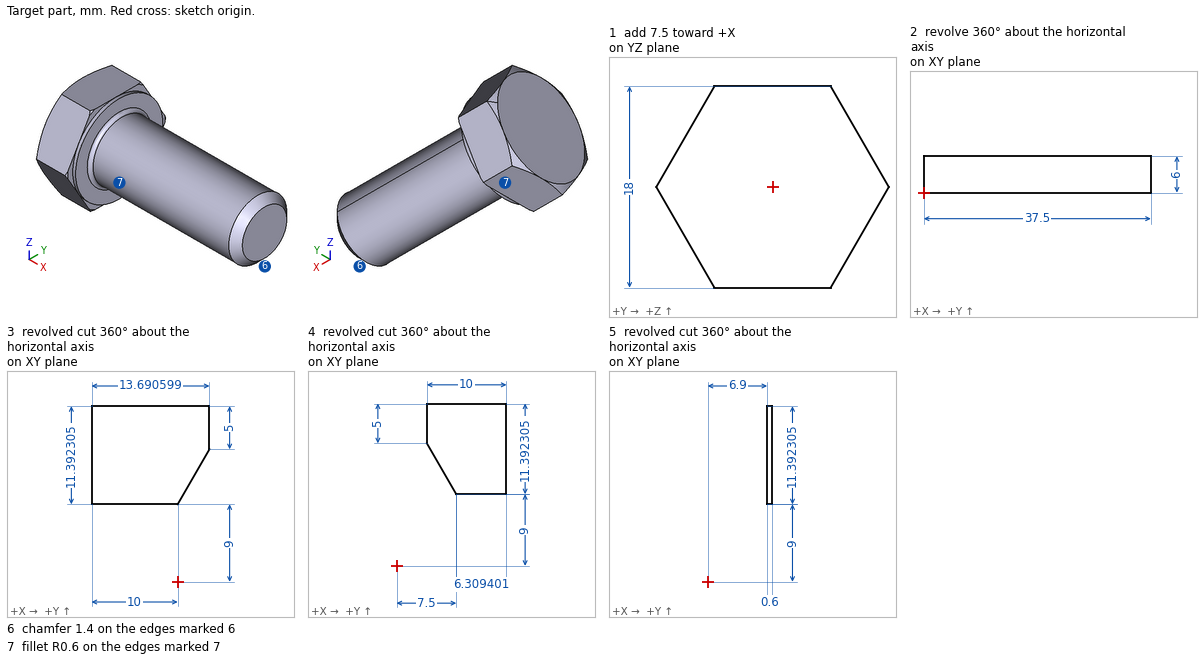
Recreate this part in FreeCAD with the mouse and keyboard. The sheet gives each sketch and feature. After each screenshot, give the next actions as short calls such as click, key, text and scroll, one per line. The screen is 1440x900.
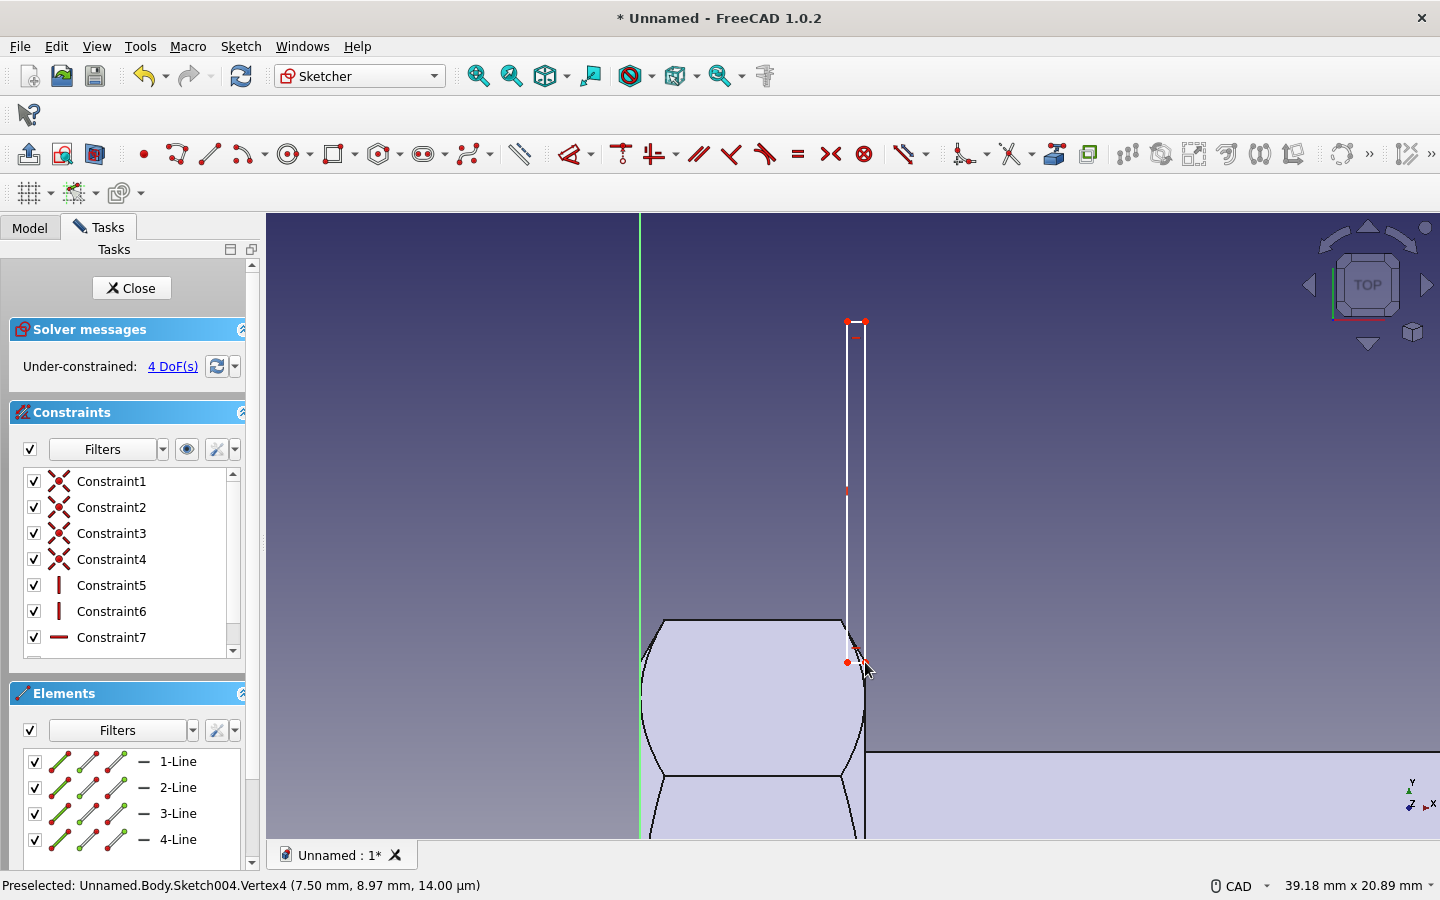
key(d)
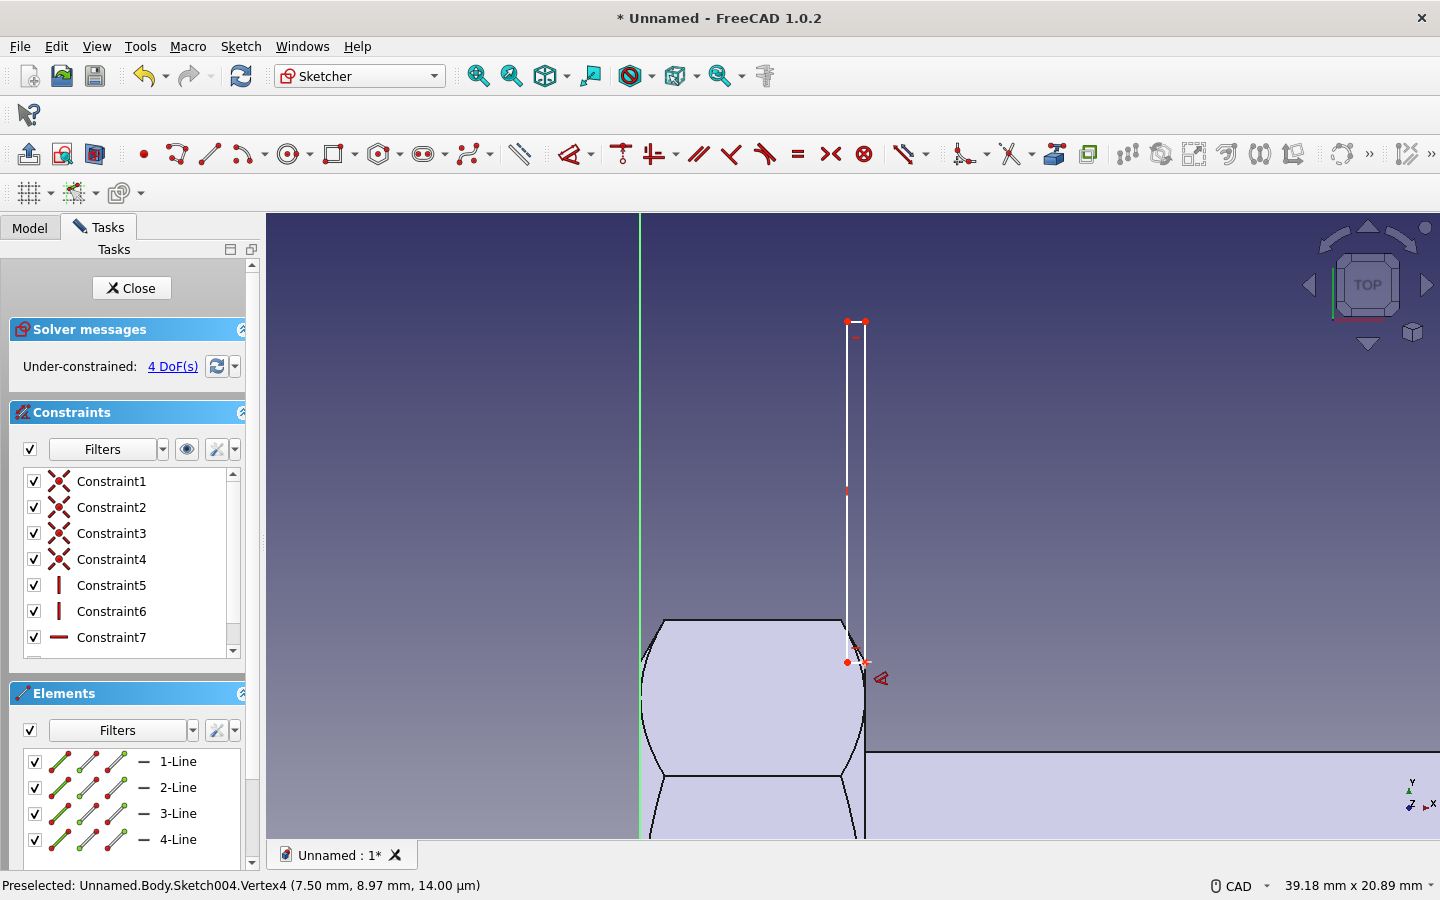
click(847, 663)
click(606, 737)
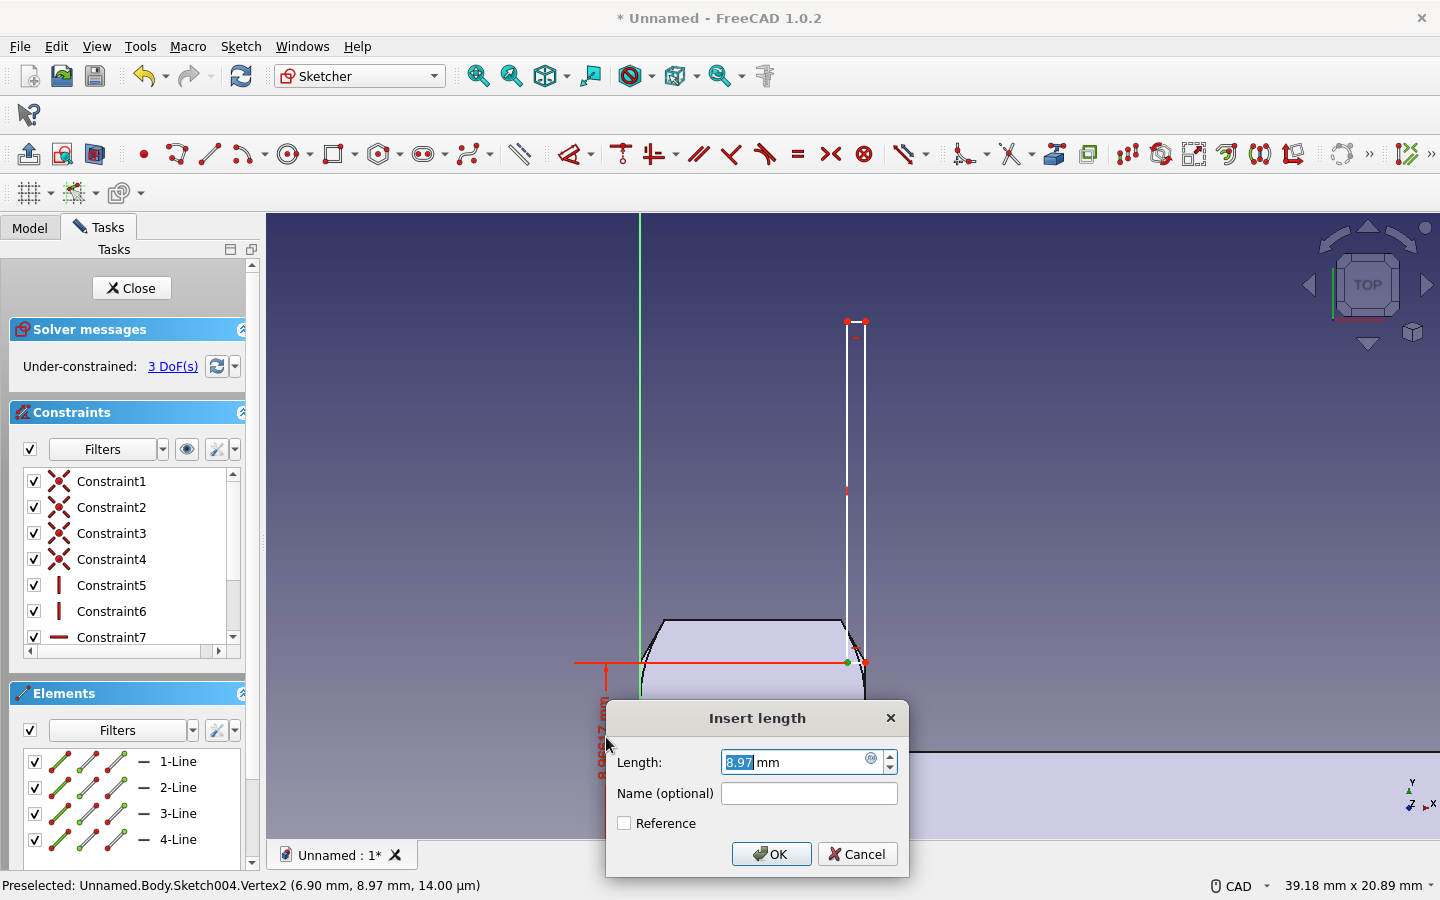
text(9)
key(Return)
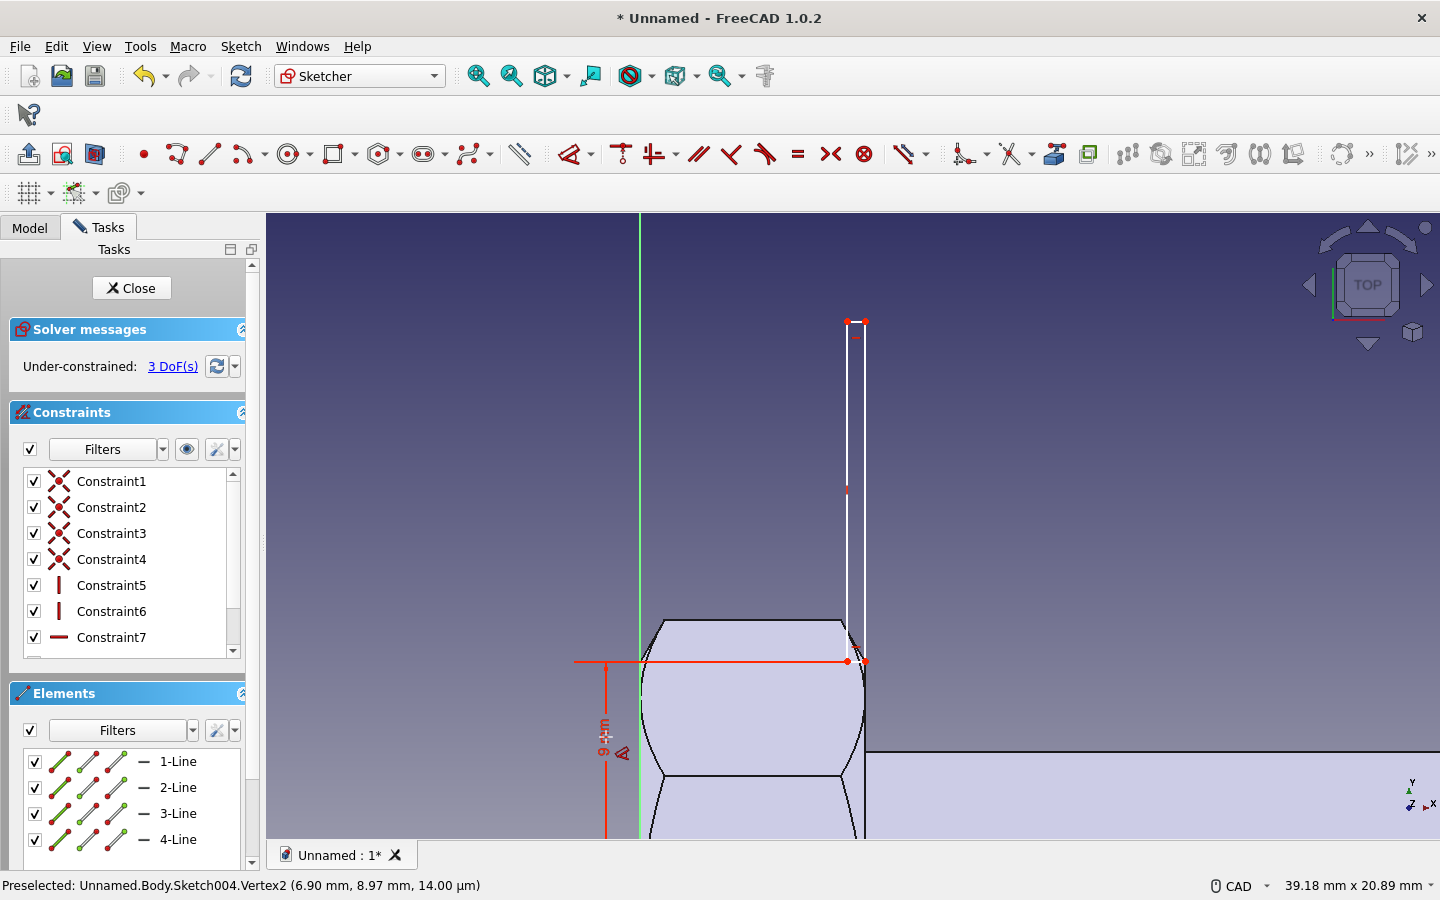
scroll(856, 662, up, 4)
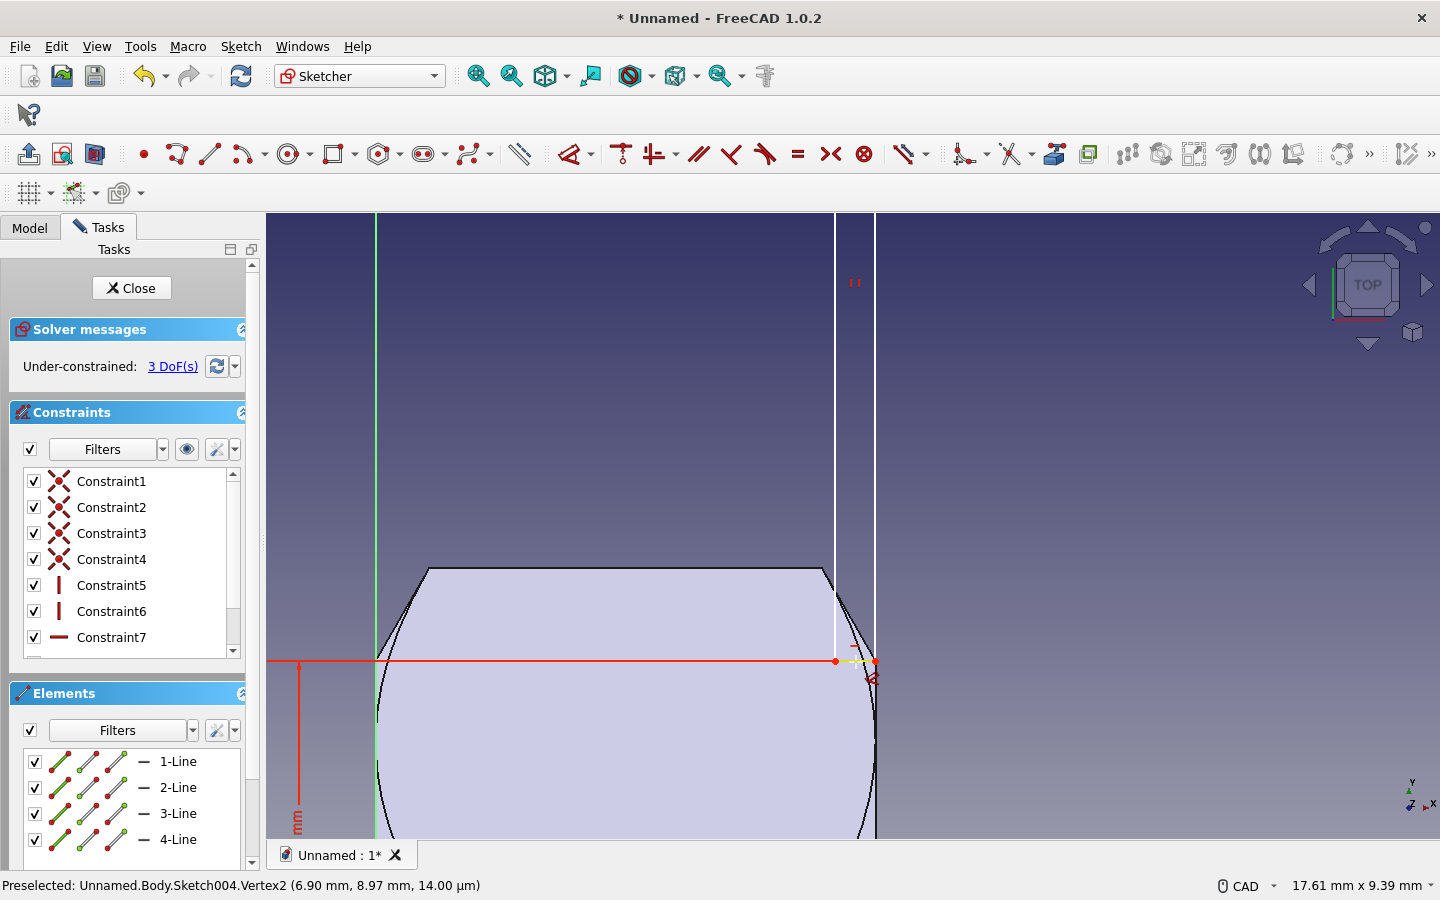
click(855, 661)
click(855, 695)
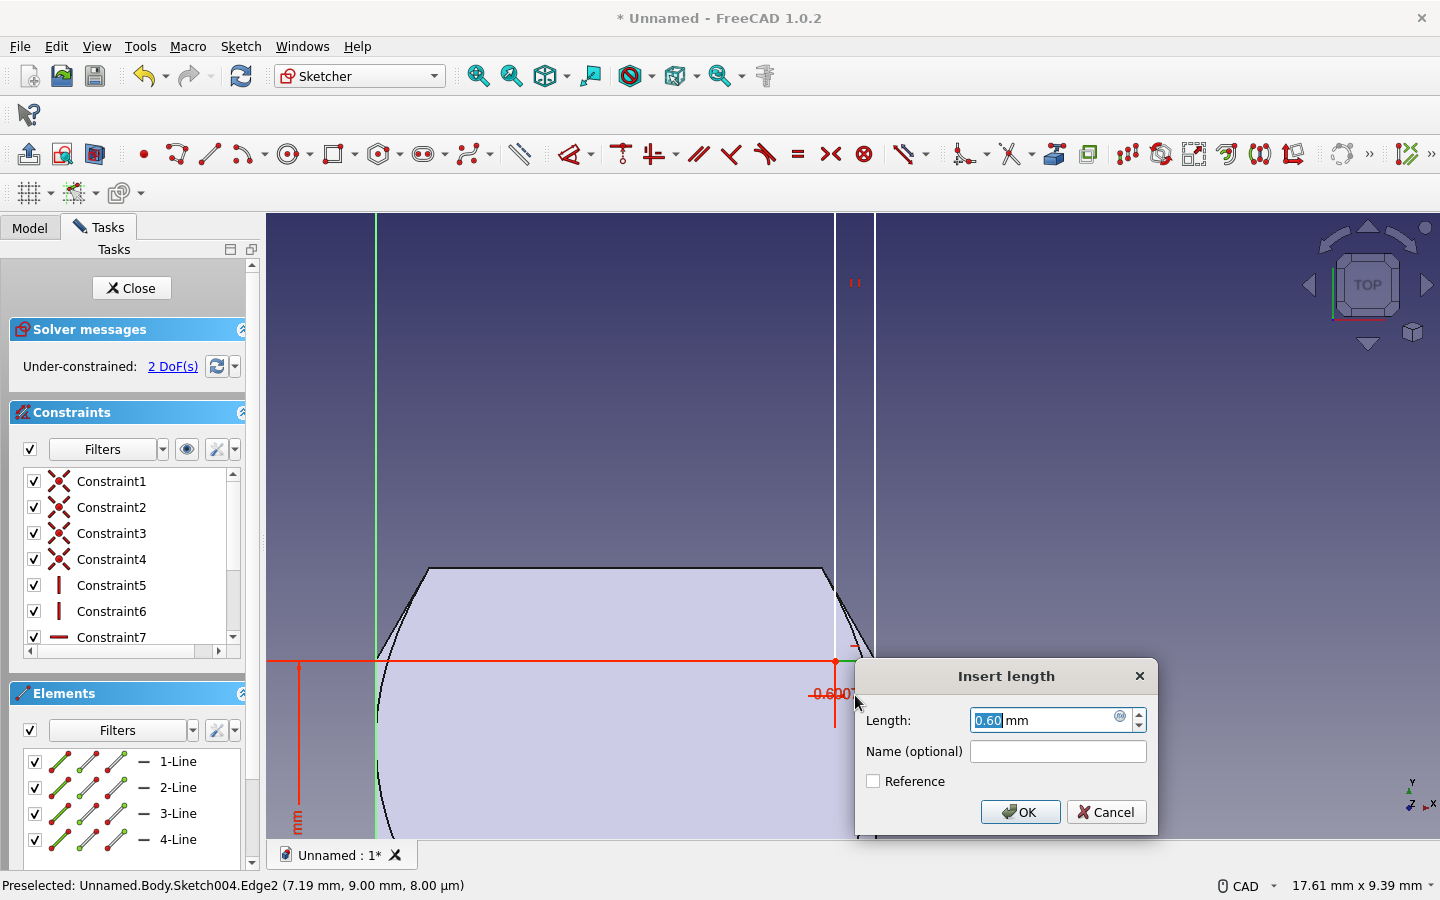
text(0.6)
key(Return)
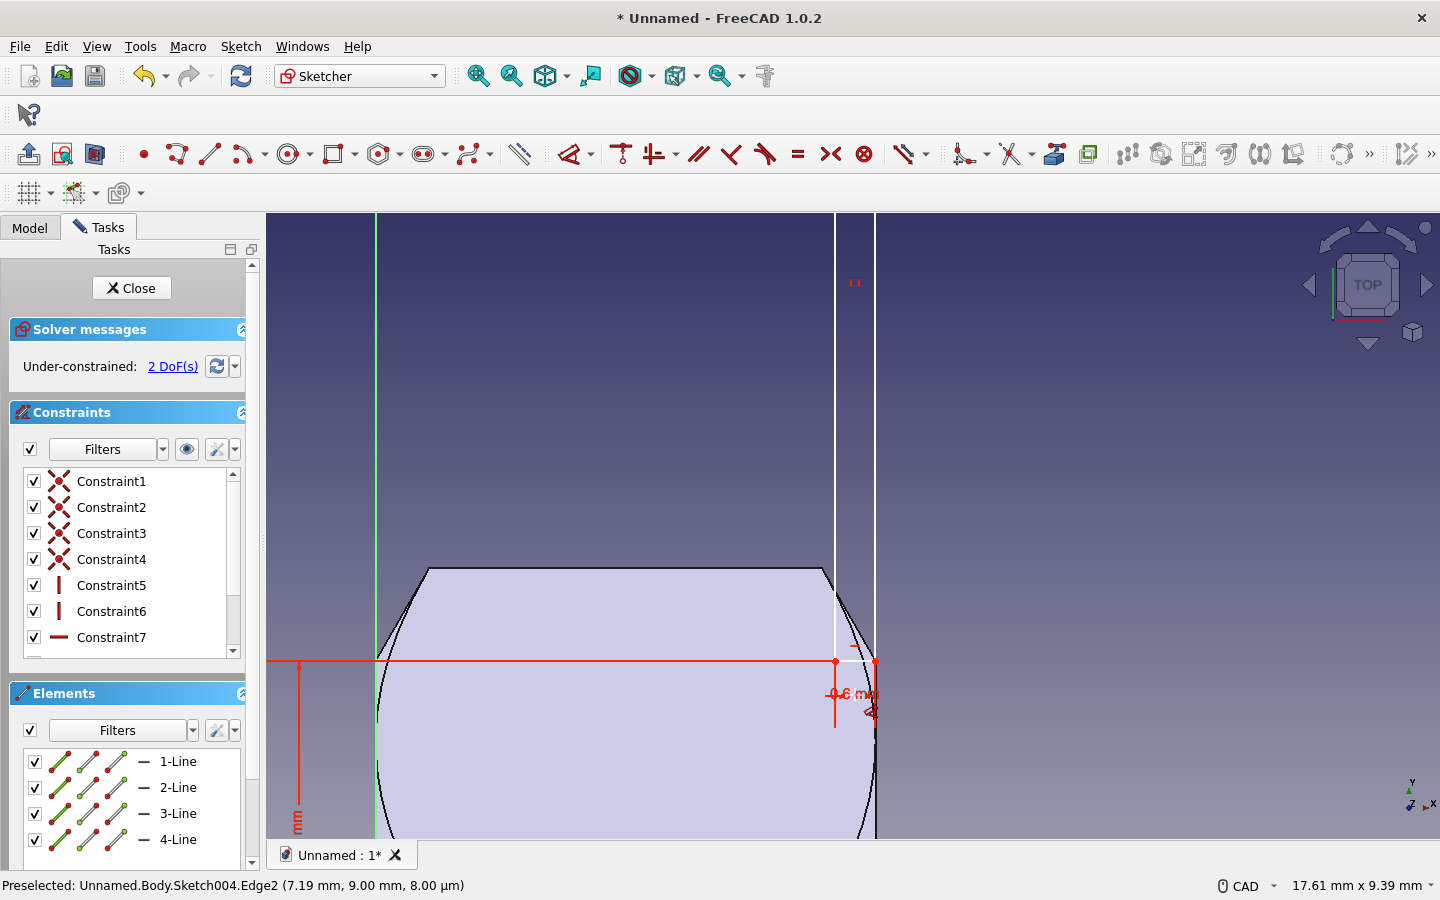
scroll(853, 502, down, 6)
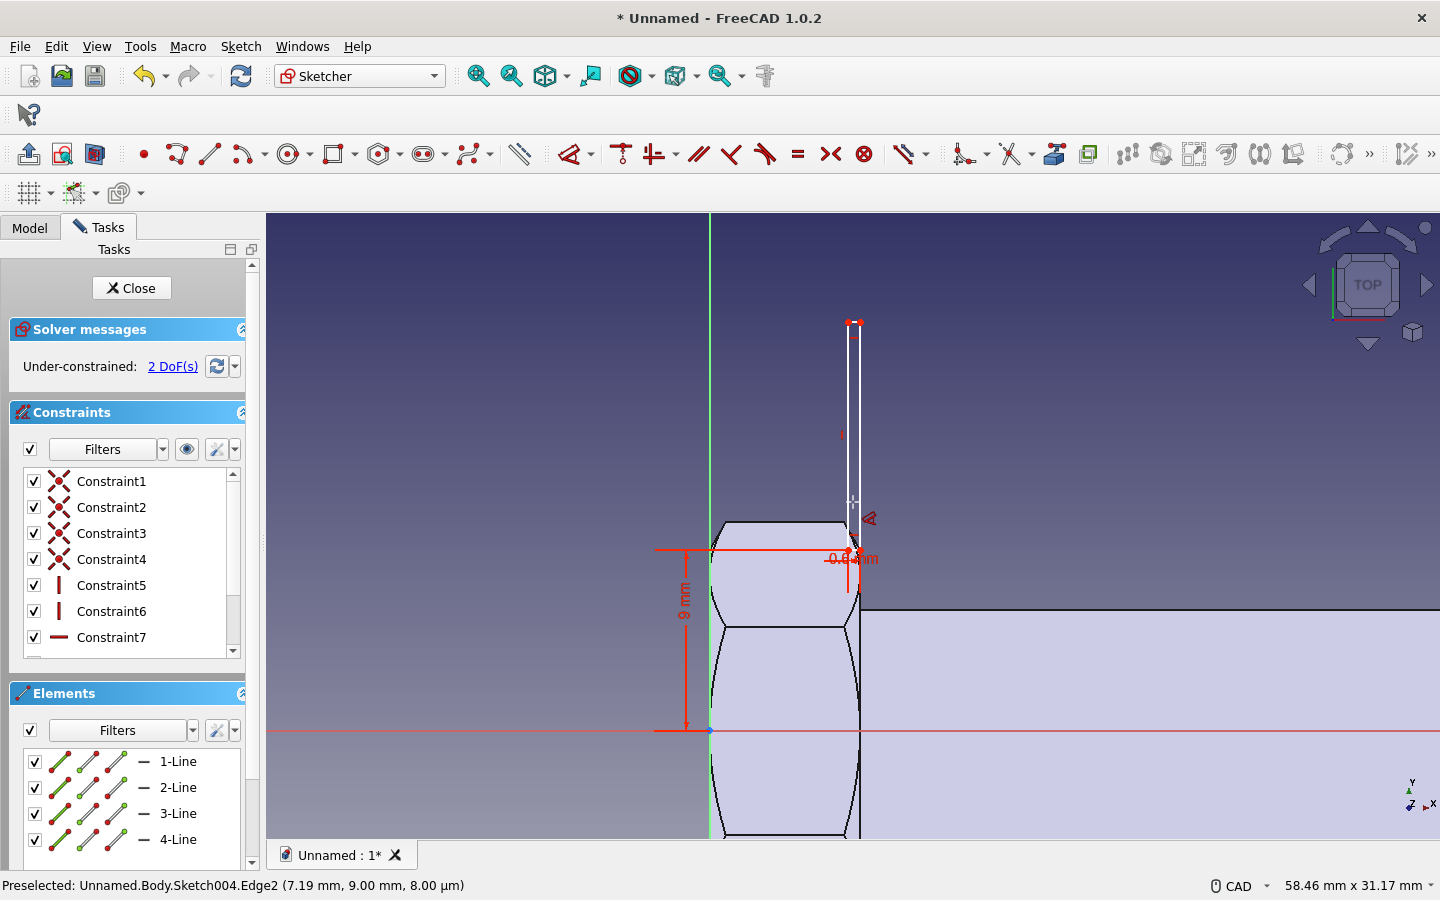
click(848, 322)
click(779, 765)